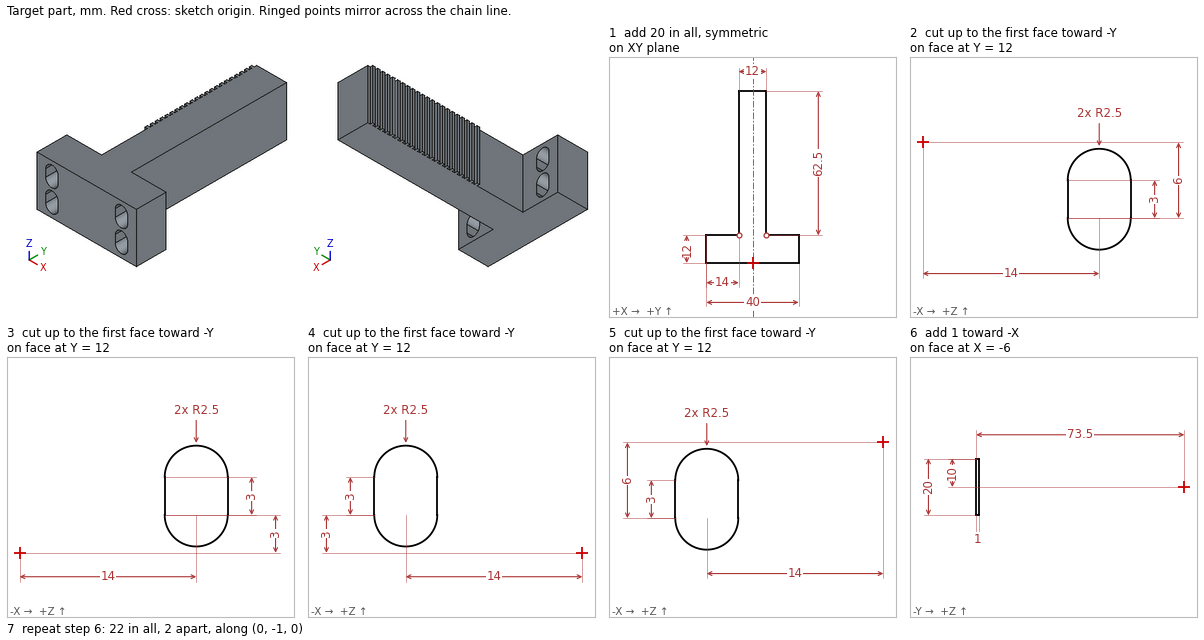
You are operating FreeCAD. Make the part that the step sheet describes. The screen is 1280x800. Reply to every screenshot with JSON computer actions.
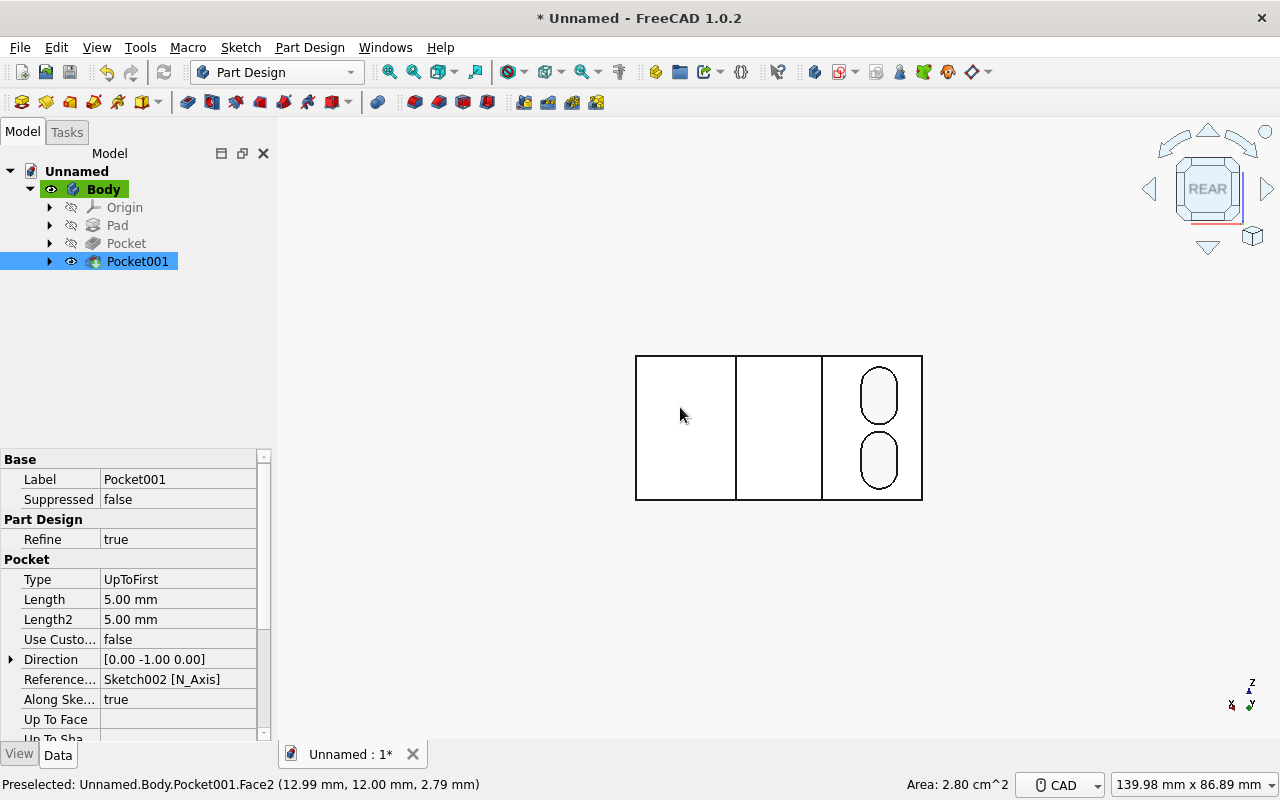
{"action": "left_click", "coordinate": [840, 72]}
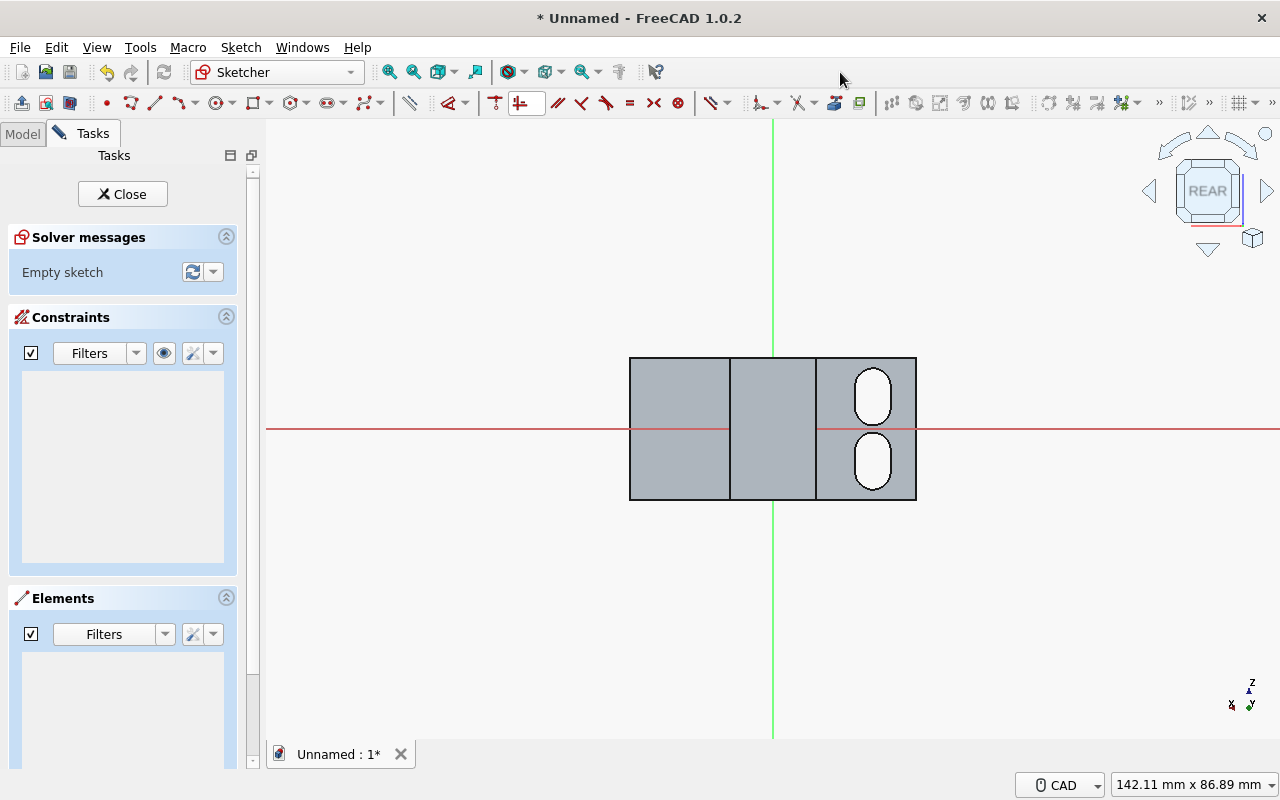
{"action": "left_click", "coordinate": [70, 104]}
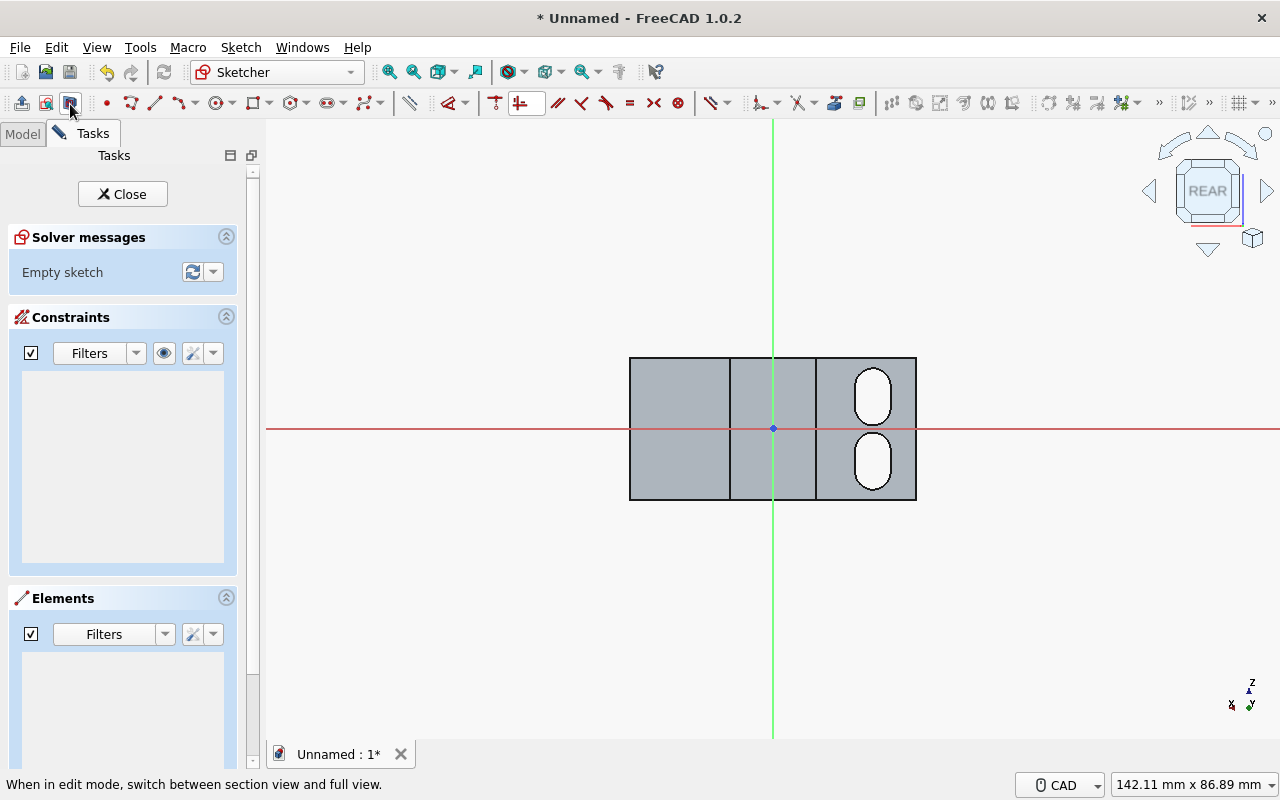
{"action": "scroll", "coordinate": [717, 391], "scroll_direction": "up", "scroll_amount": 8}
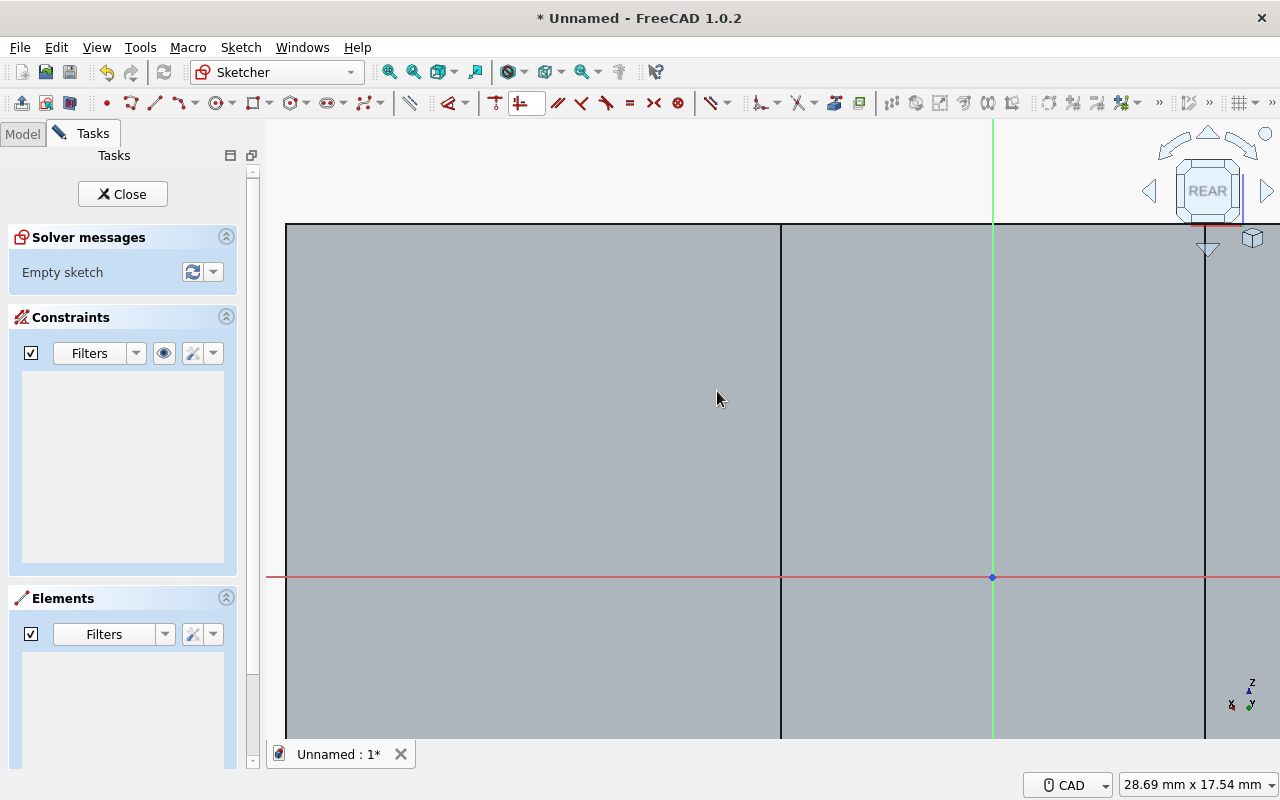
{"action": "left_click", "coordinate": [328, 104]}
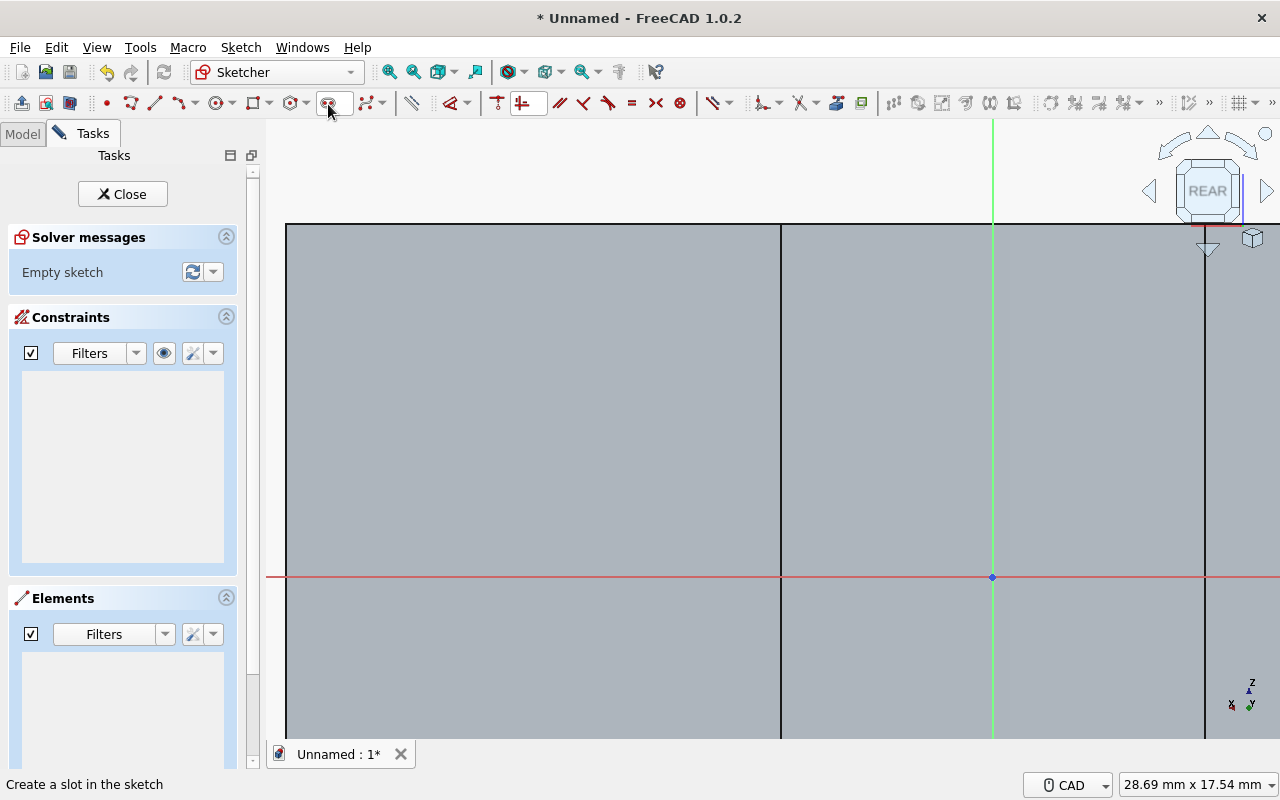
{"action": "left_click", "coordinate": [498, 471]}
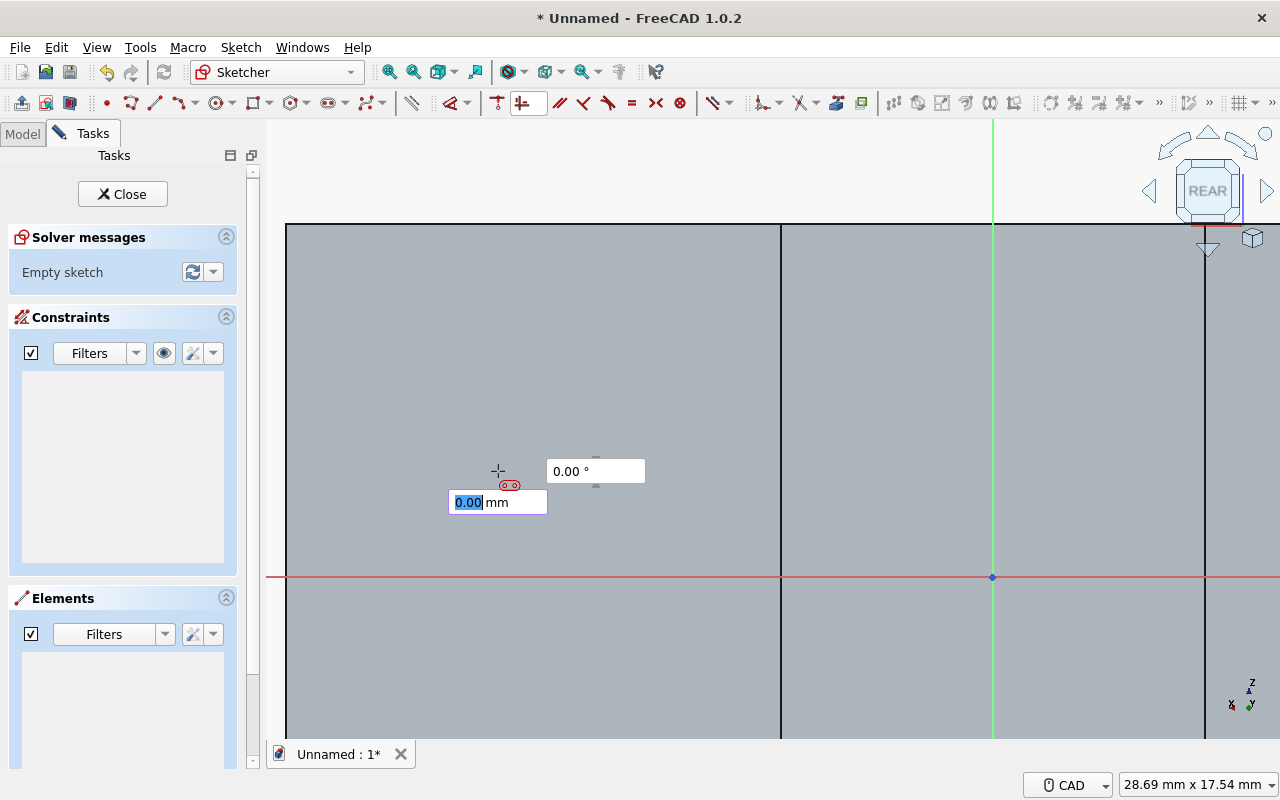
{"action": "left_click", "coordinate": [498, 365]}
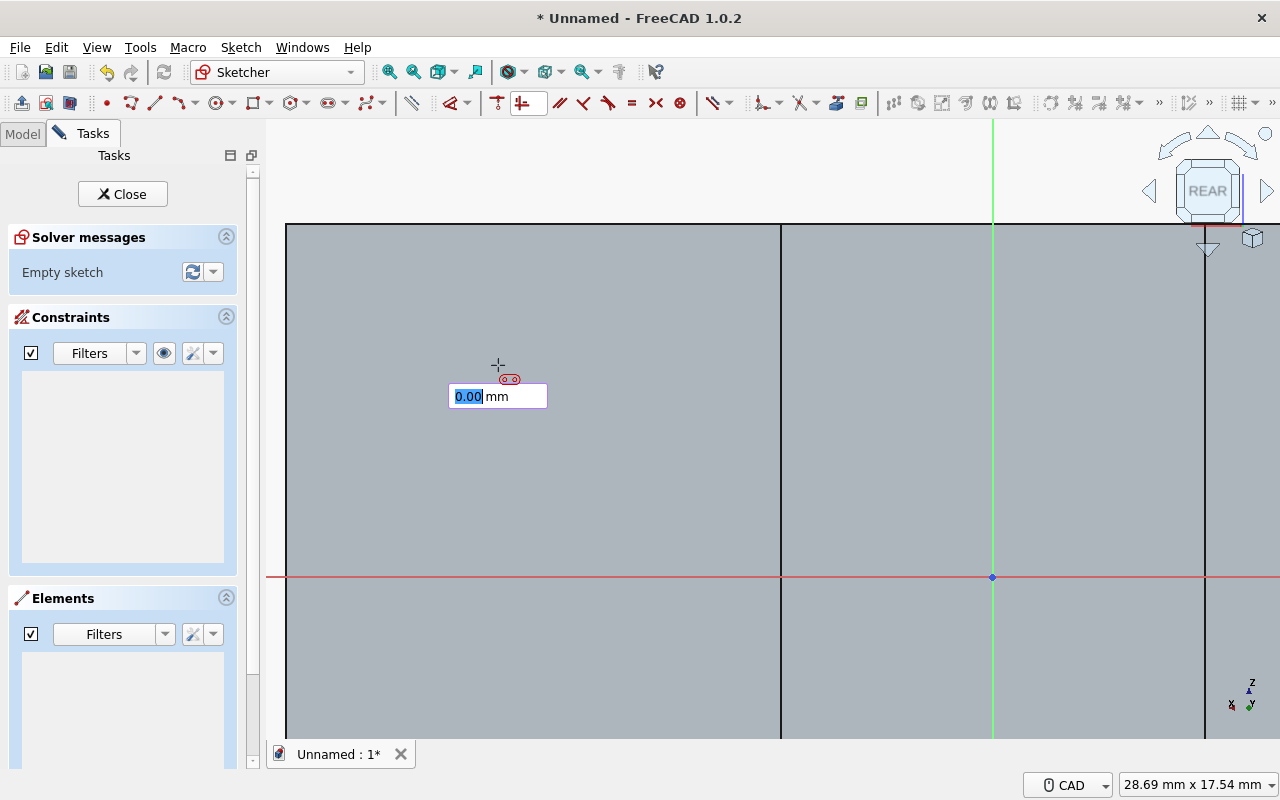
{"action": "left_click", "coordinate": [409, 418]}
{"action": "key", "text": "Escape"}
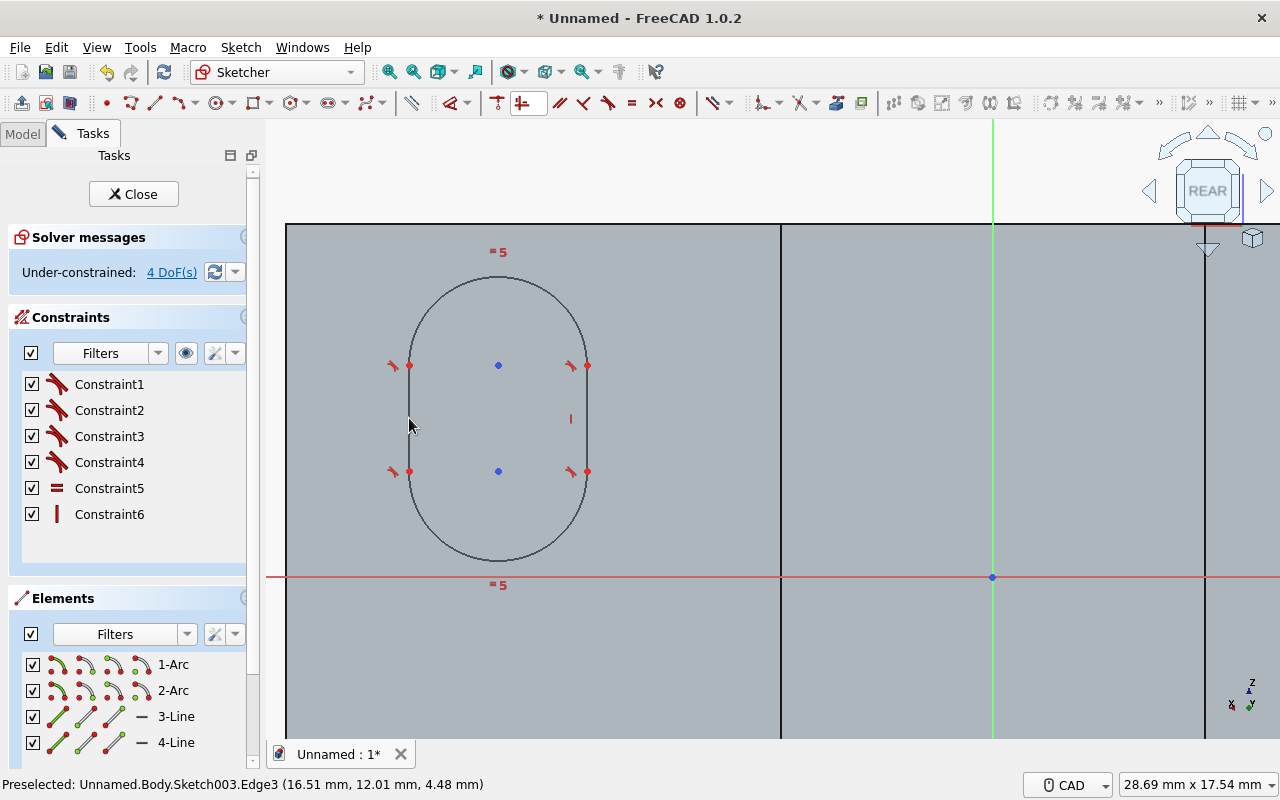
{"action": "left_click", "coordinate": [450, 104]}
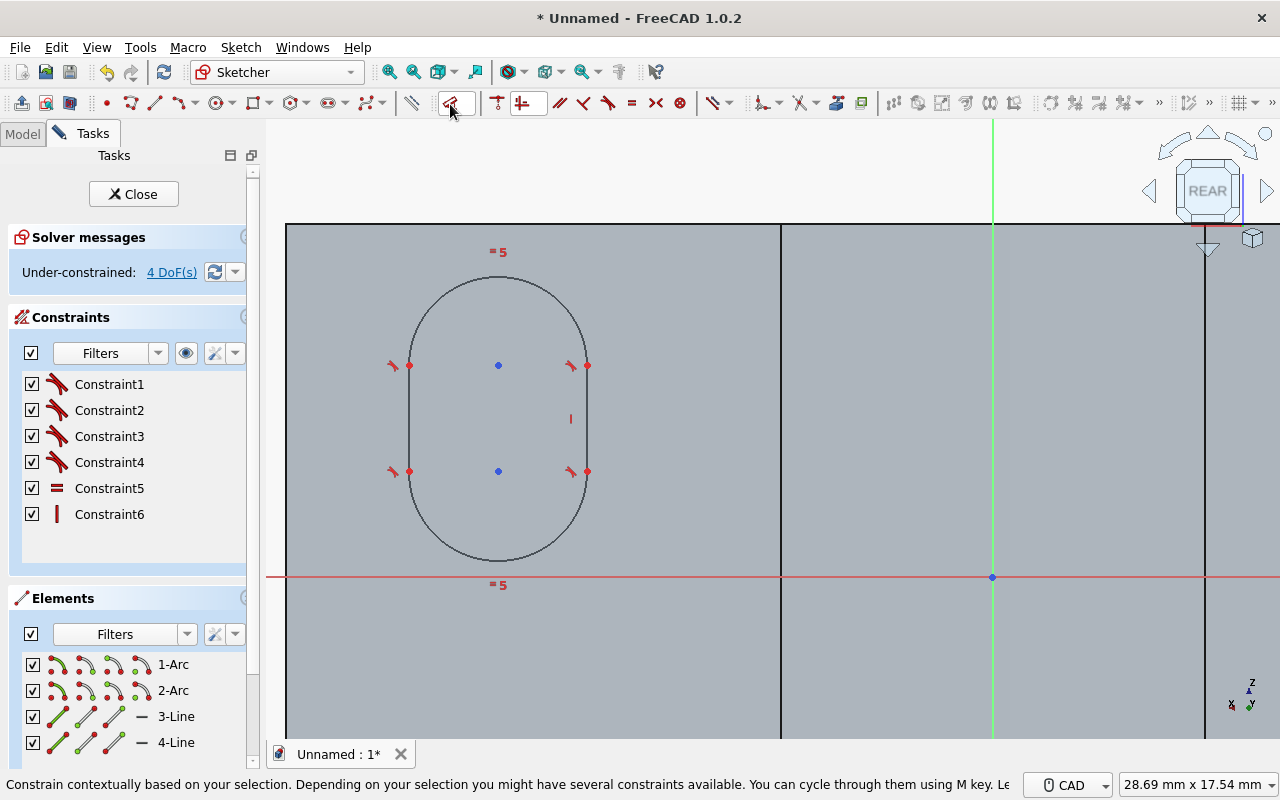
{"action": "left_click", "coordinate": [446, 544]}
{"action": "left_click", "coordinate": [389, 524]}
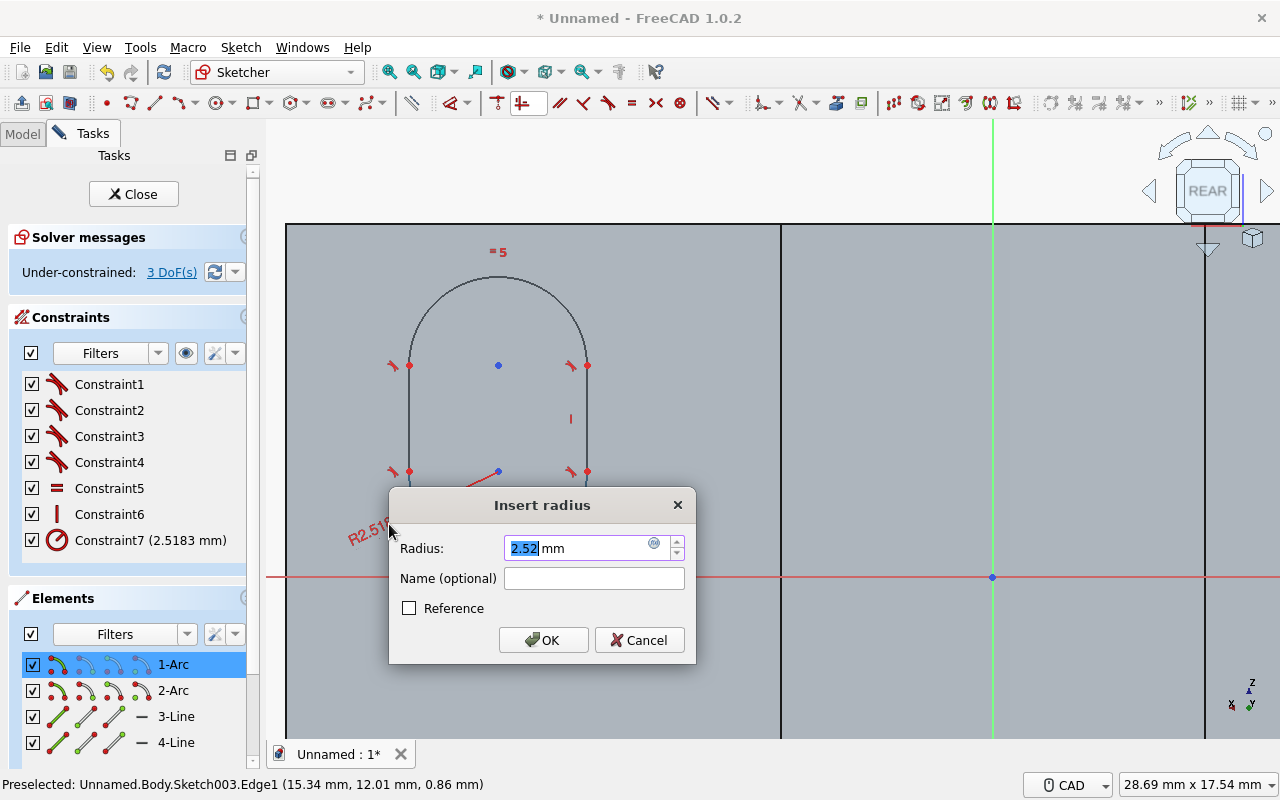
{"action": "type", "text": "2.5"}
{"action": "key", "text": "Return"}